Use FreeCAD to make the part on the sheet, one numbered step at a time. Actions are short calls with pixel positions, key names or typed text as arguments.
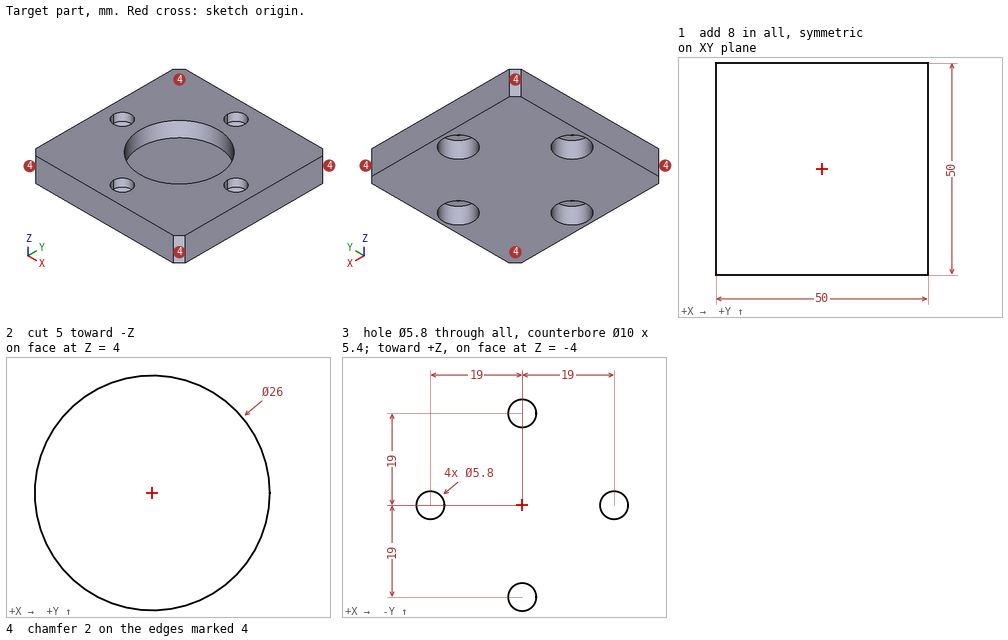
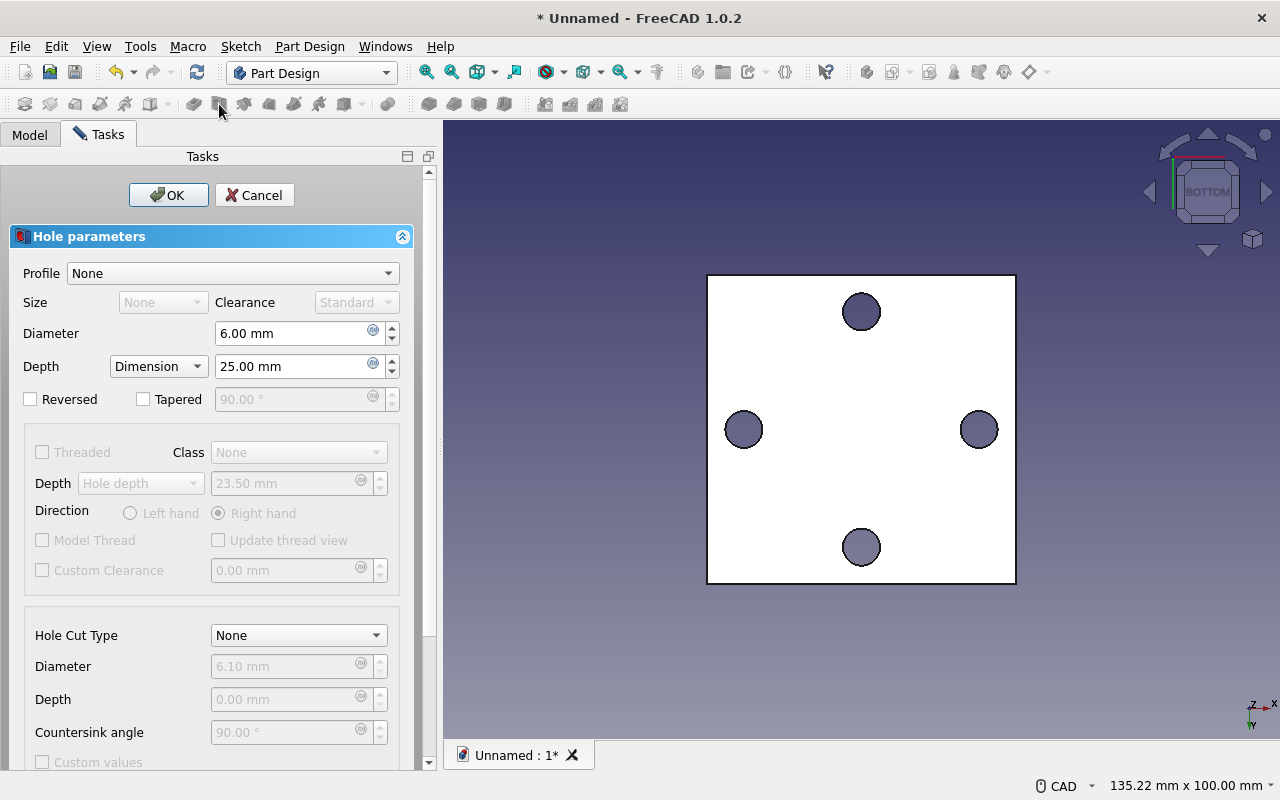
triple_click(300, 334)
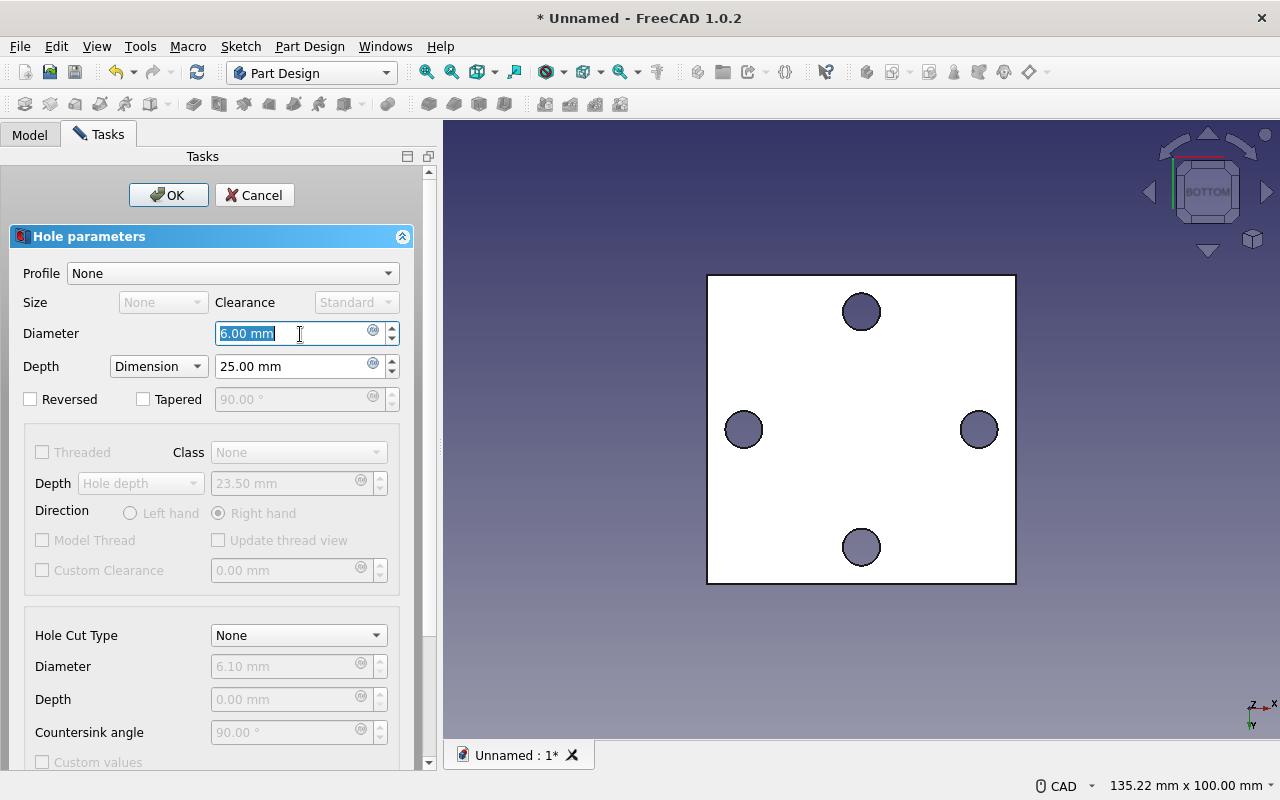
text(5.8)
key(Tab)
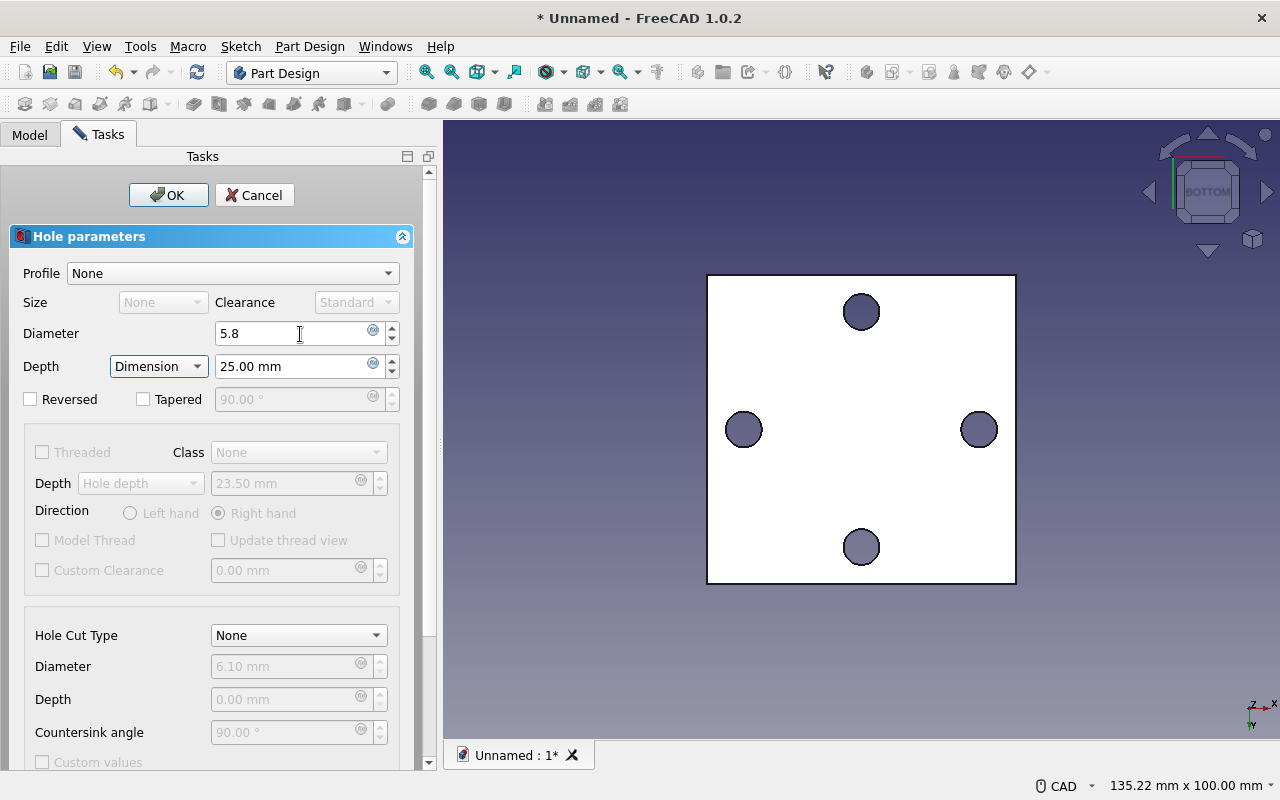
click(160, 366)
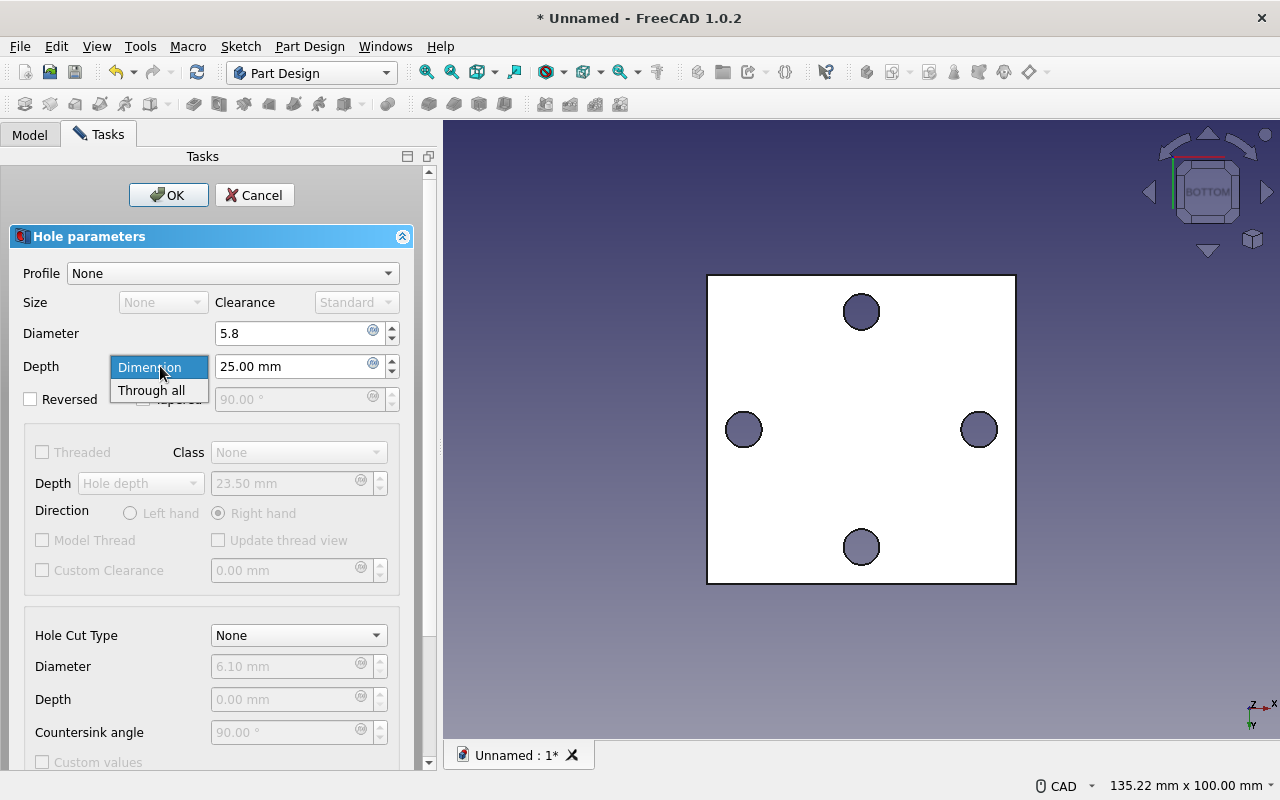
click(158, 390)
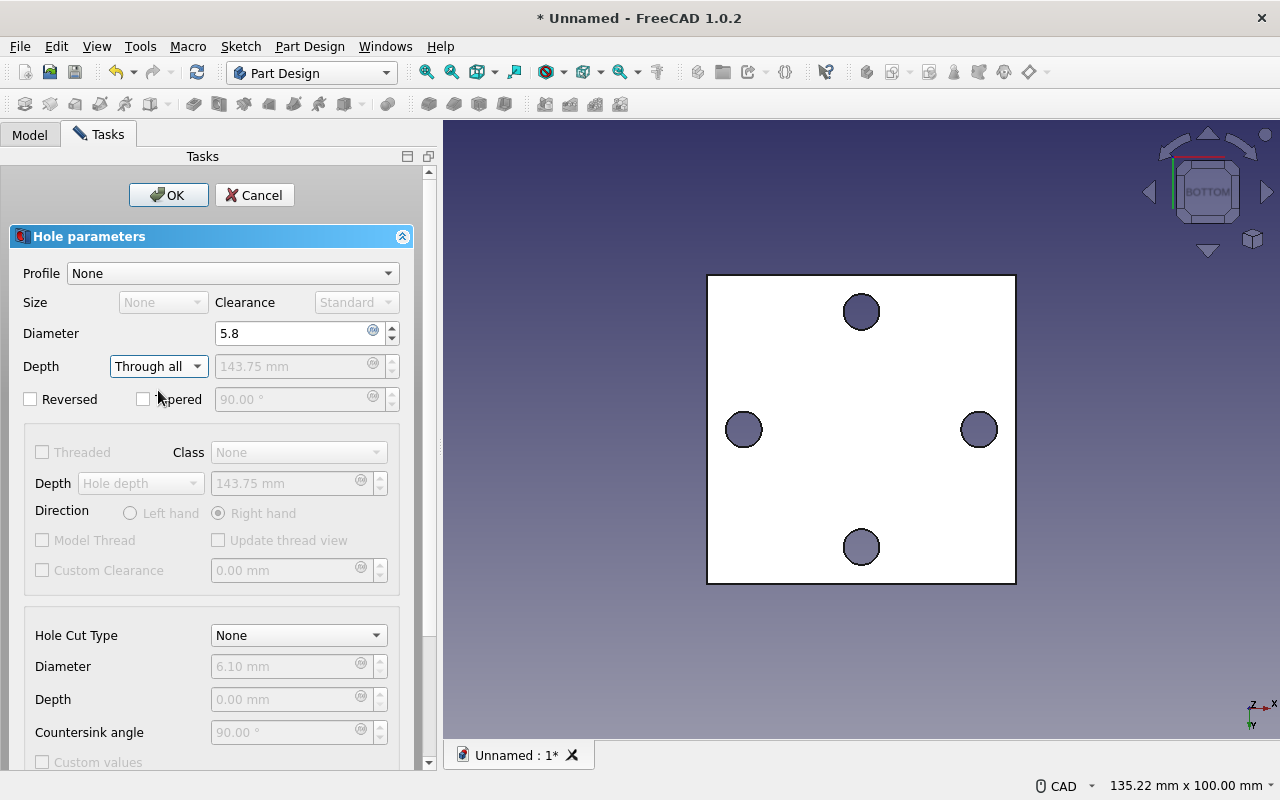
click(300, 636)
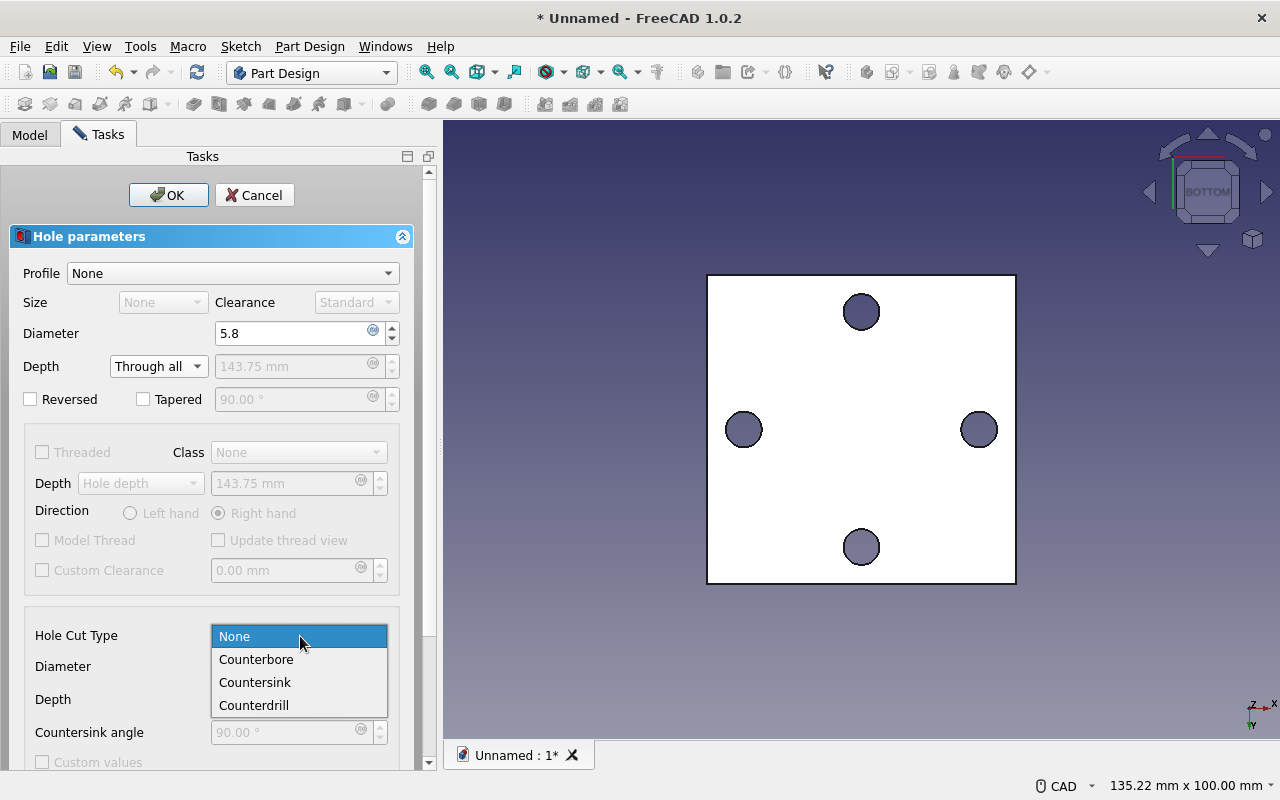
click(298, 660)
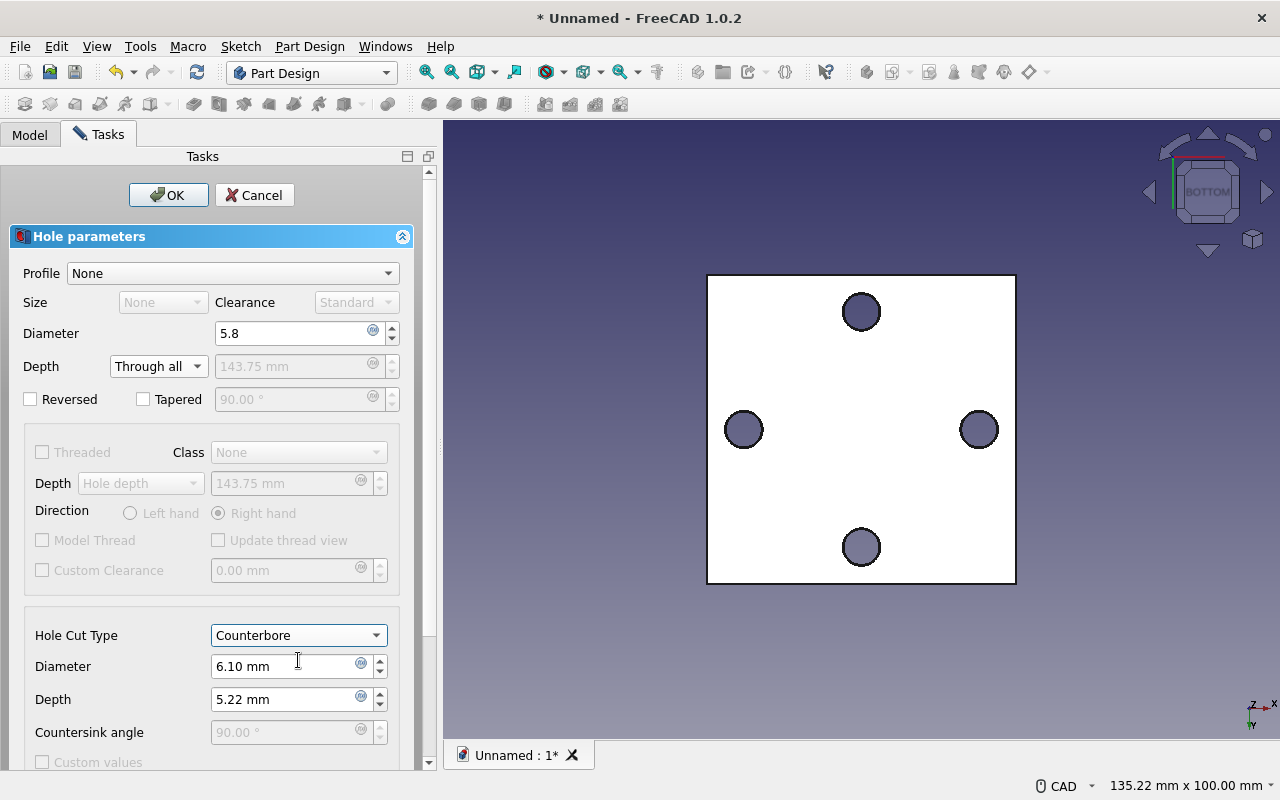
triple_click(292, 666)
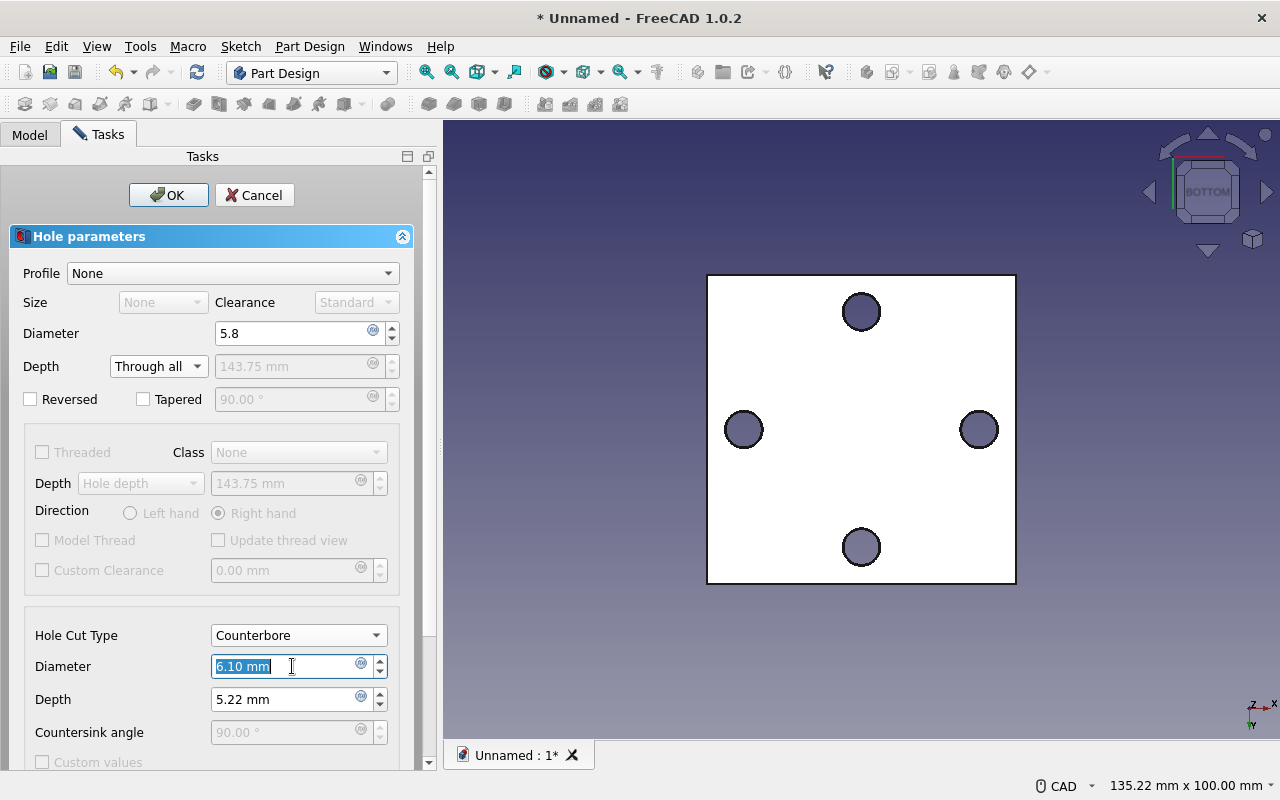
text(10)
key(Tab)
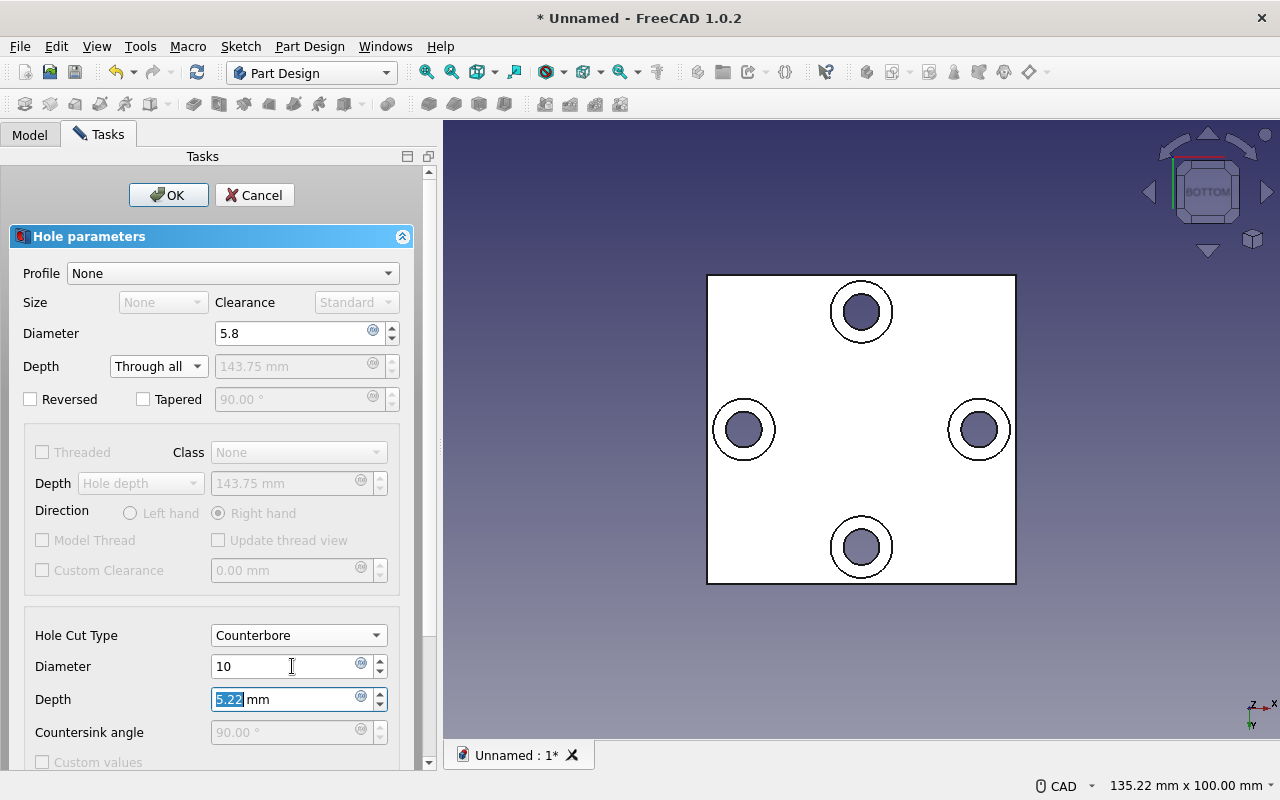
text(5.4)
key(Tab)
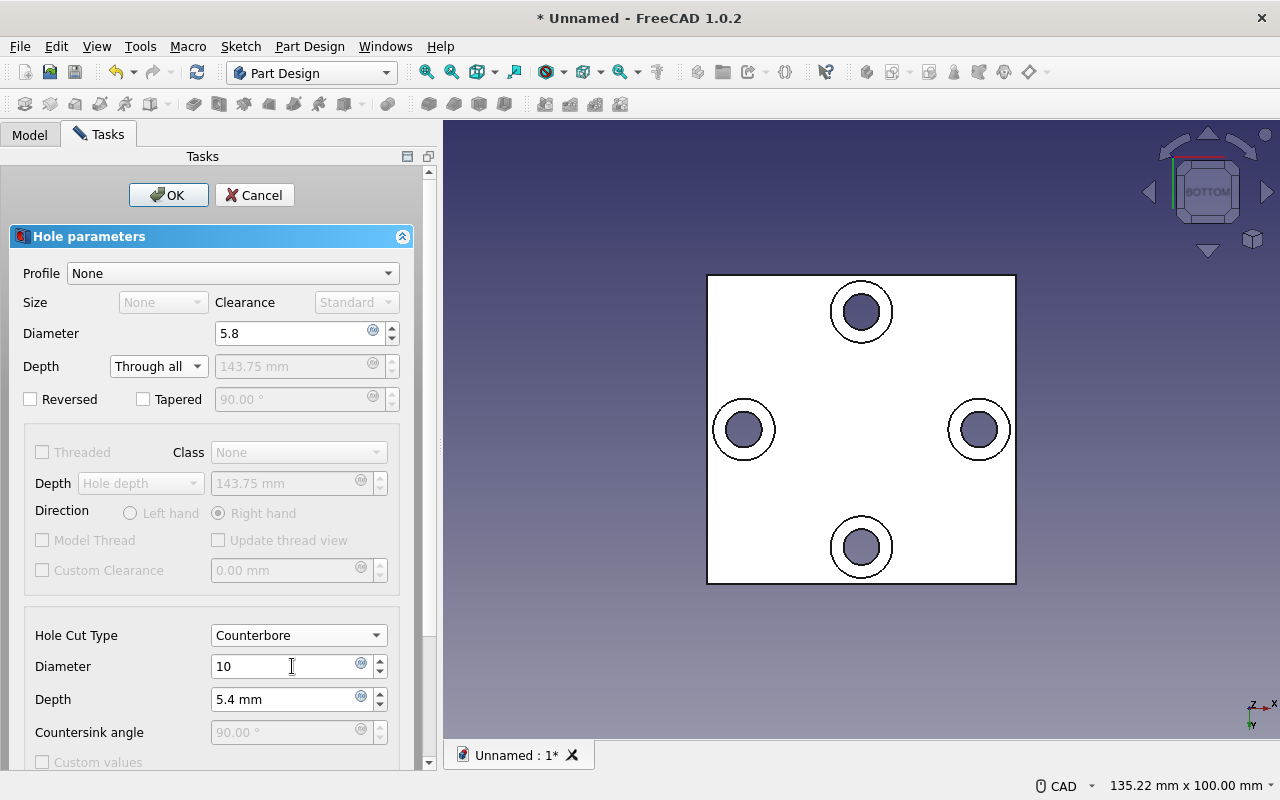
click(169, 195)